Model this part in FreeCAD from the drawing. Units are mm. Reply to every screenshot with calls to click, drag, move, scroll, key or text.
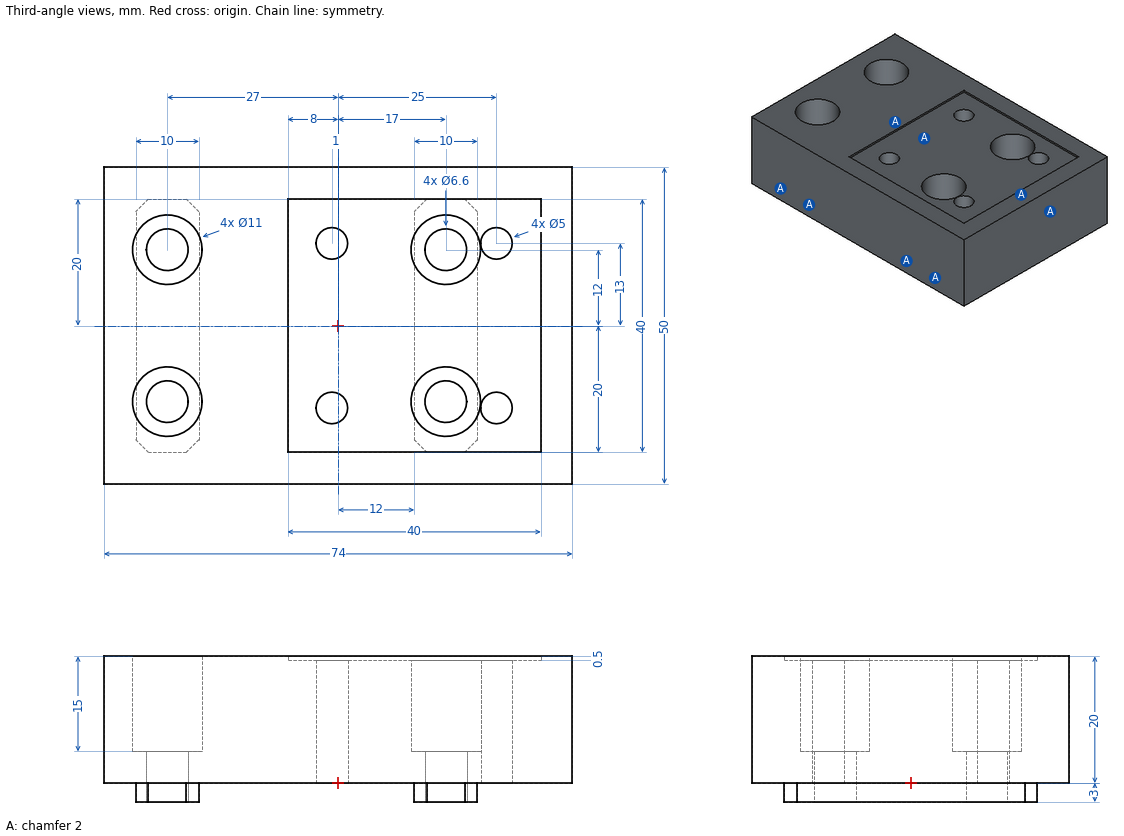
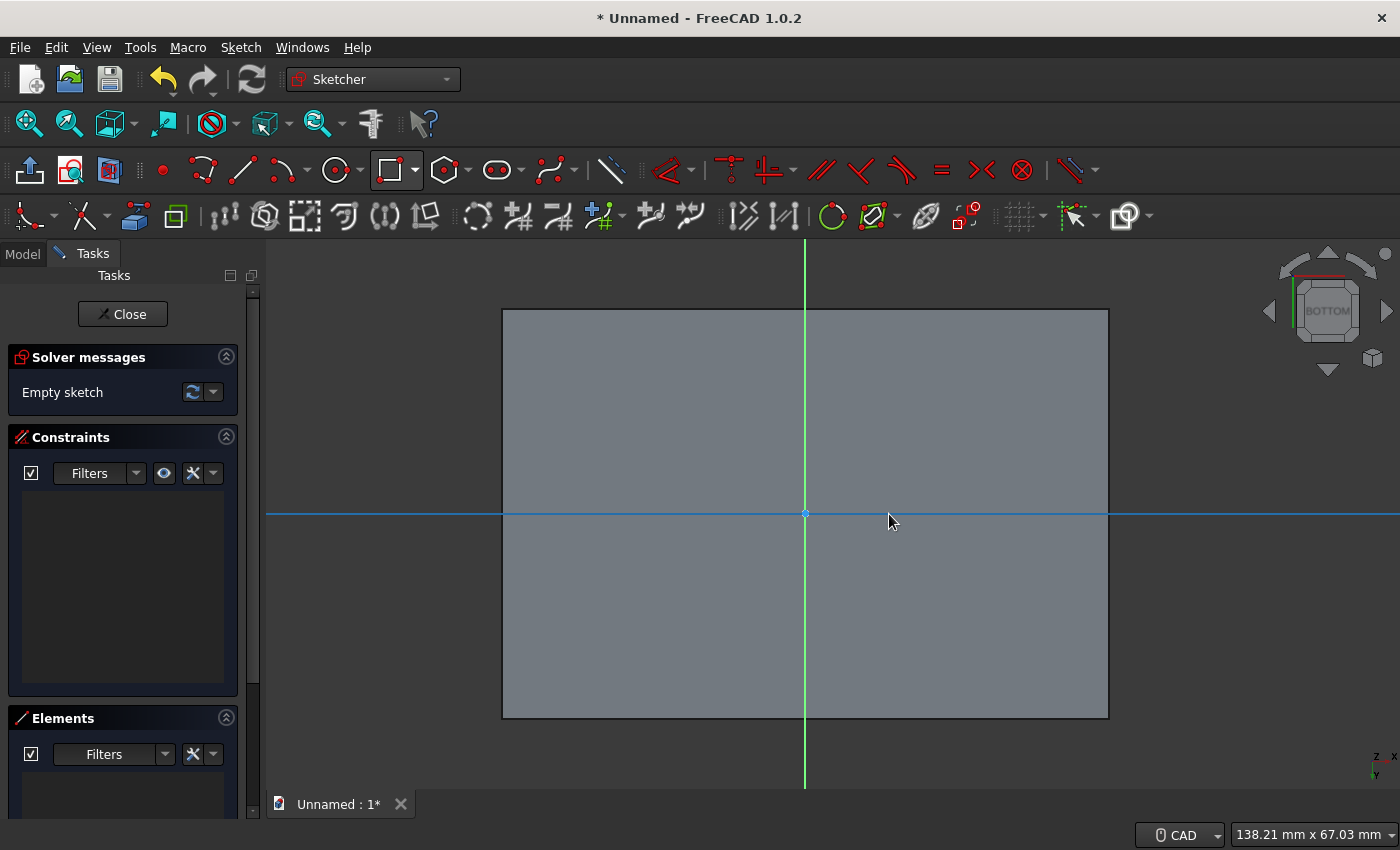
click(390, 170)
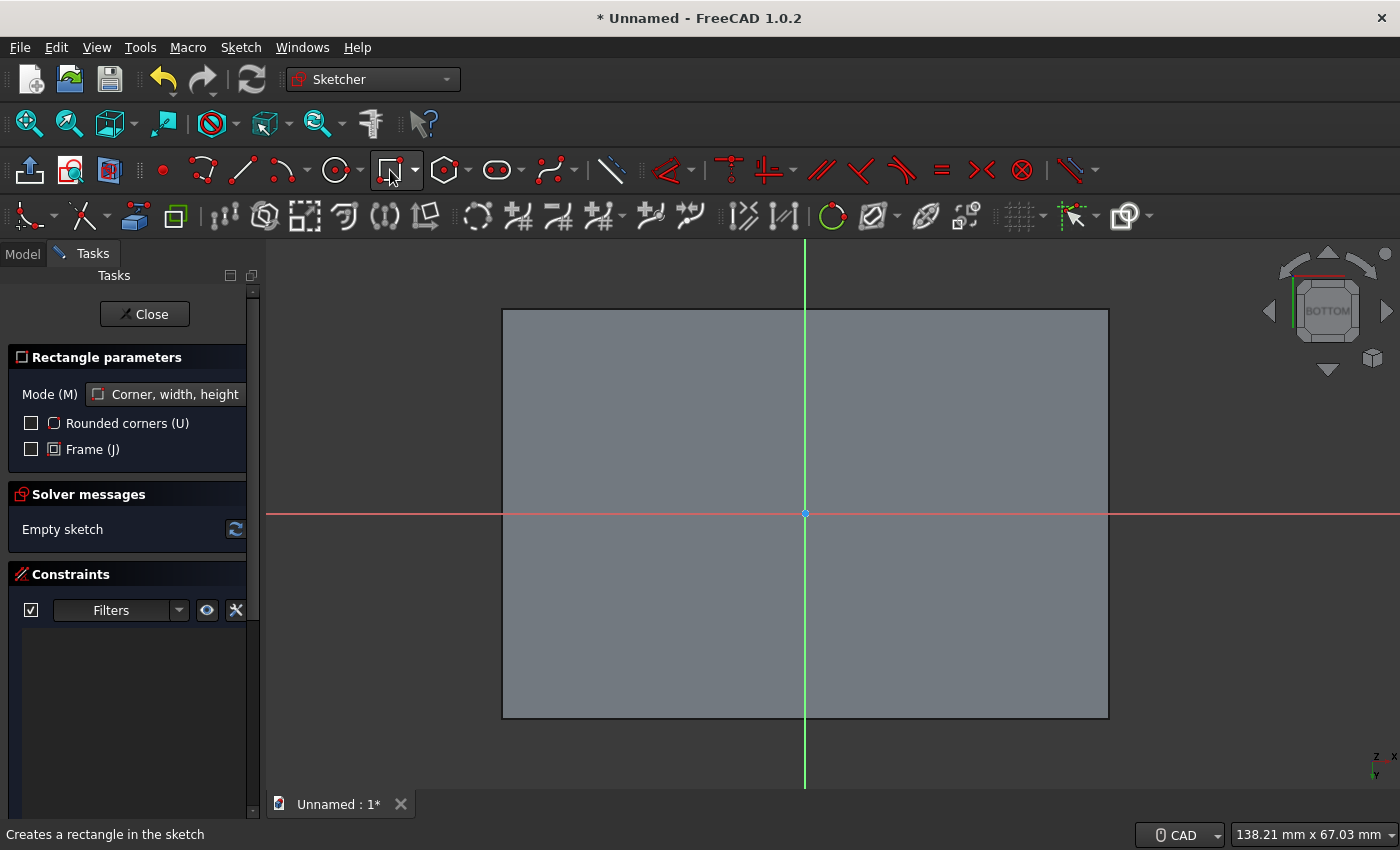
click(904, 350)
move(986, 678)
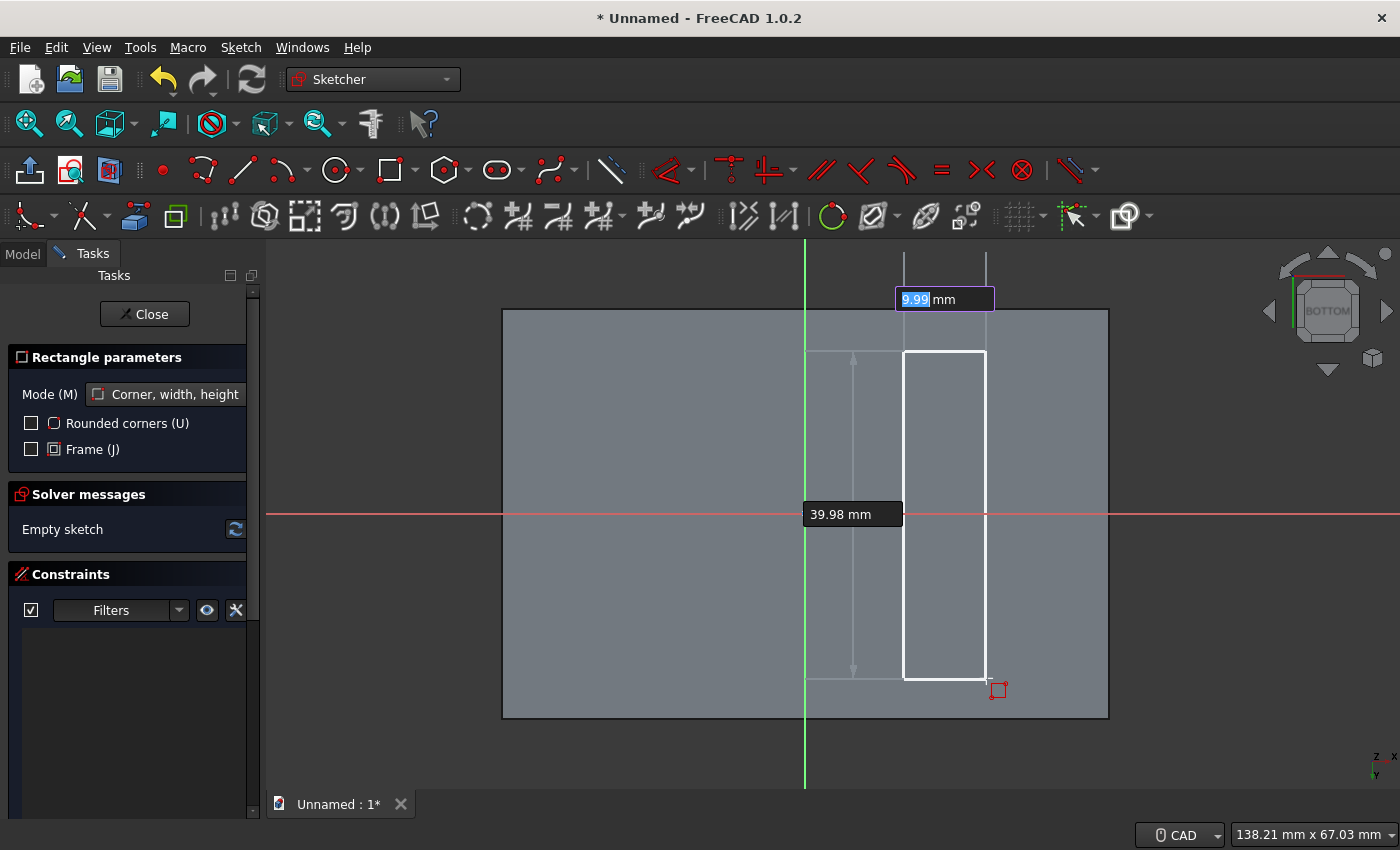
text(10)
key(Tab)
text(40)
key(Return)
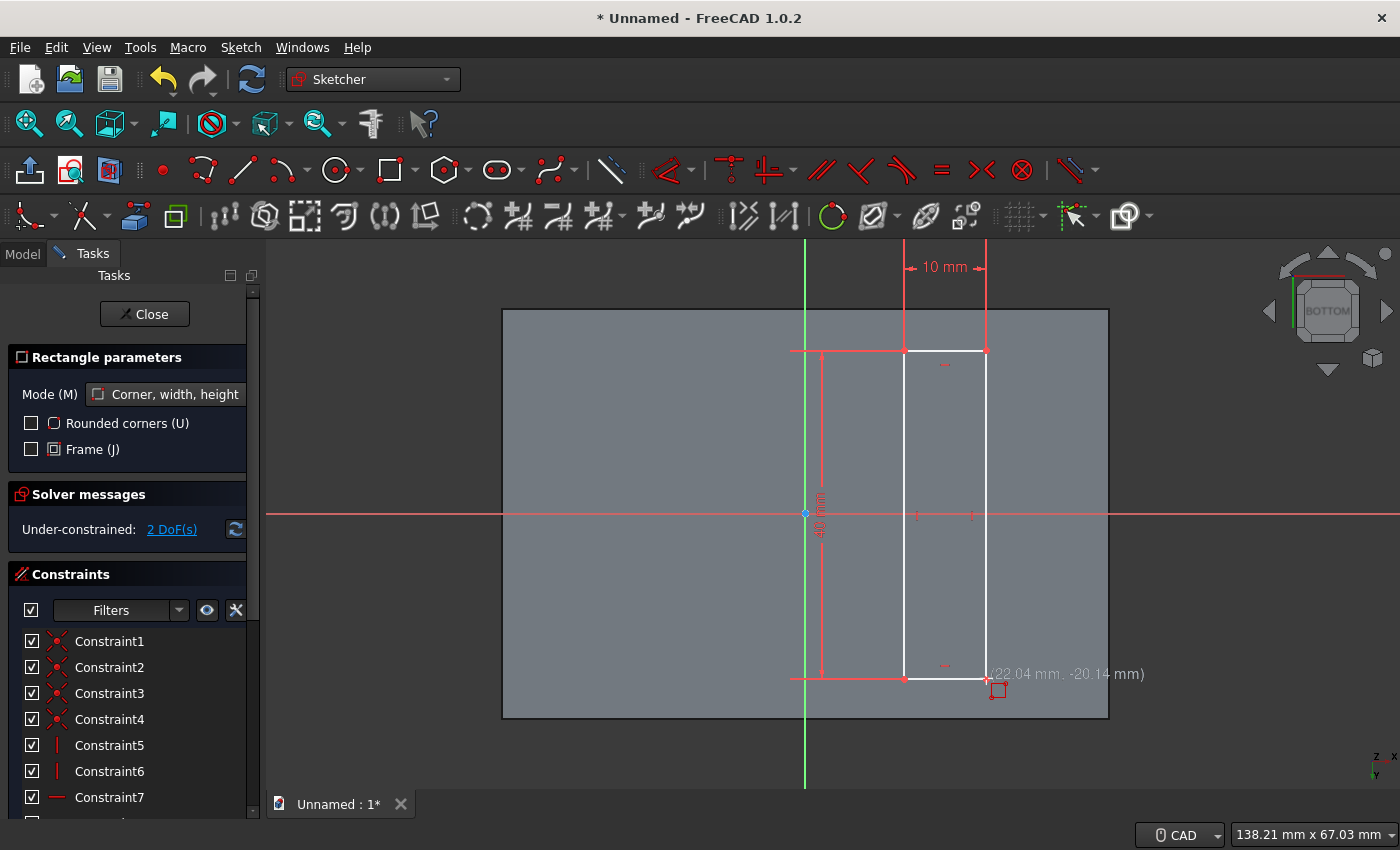
click(543, 350)
move(625, 678)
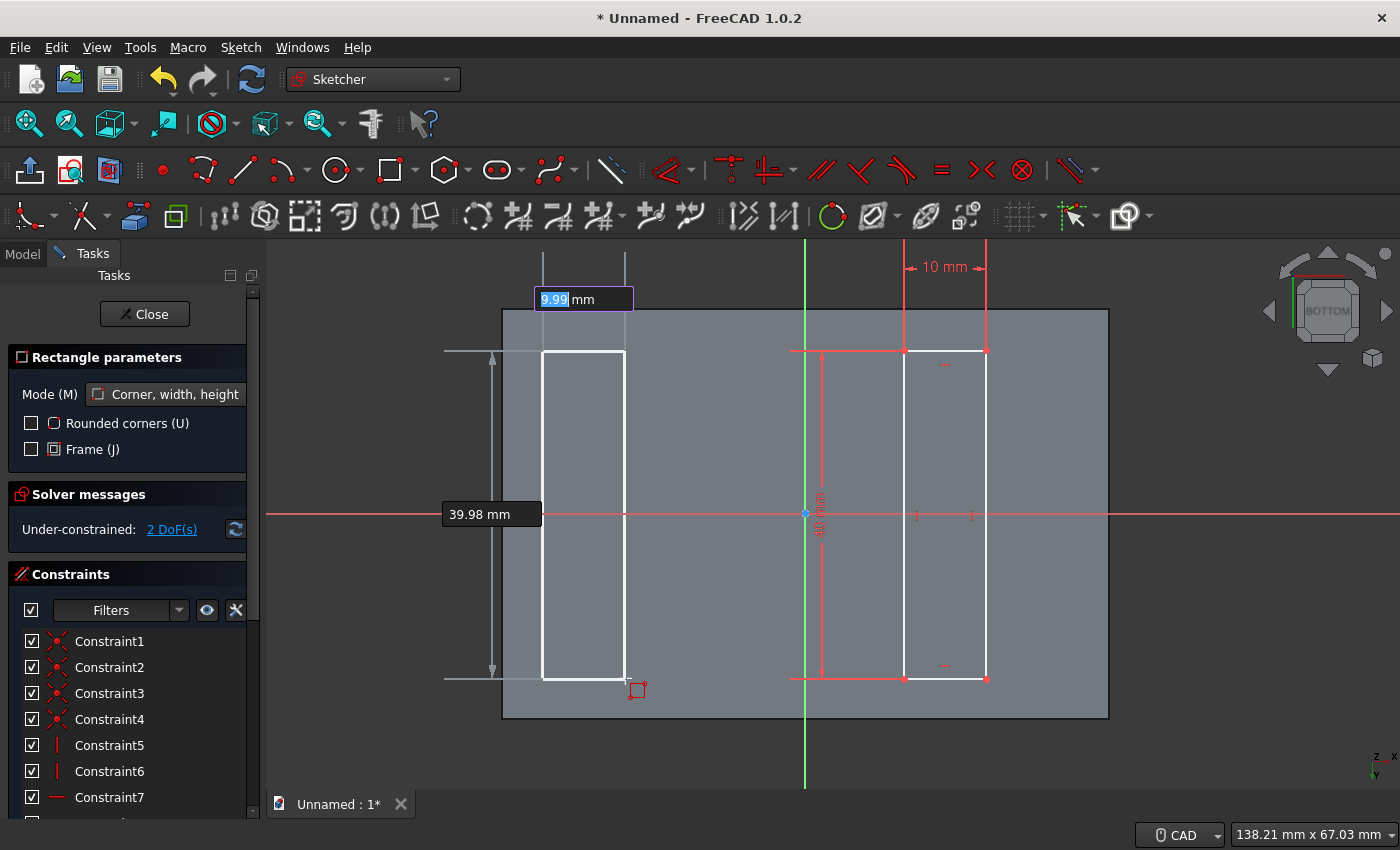
text(10)
key(Tab)
text(40)
key(Return)
key(Escape)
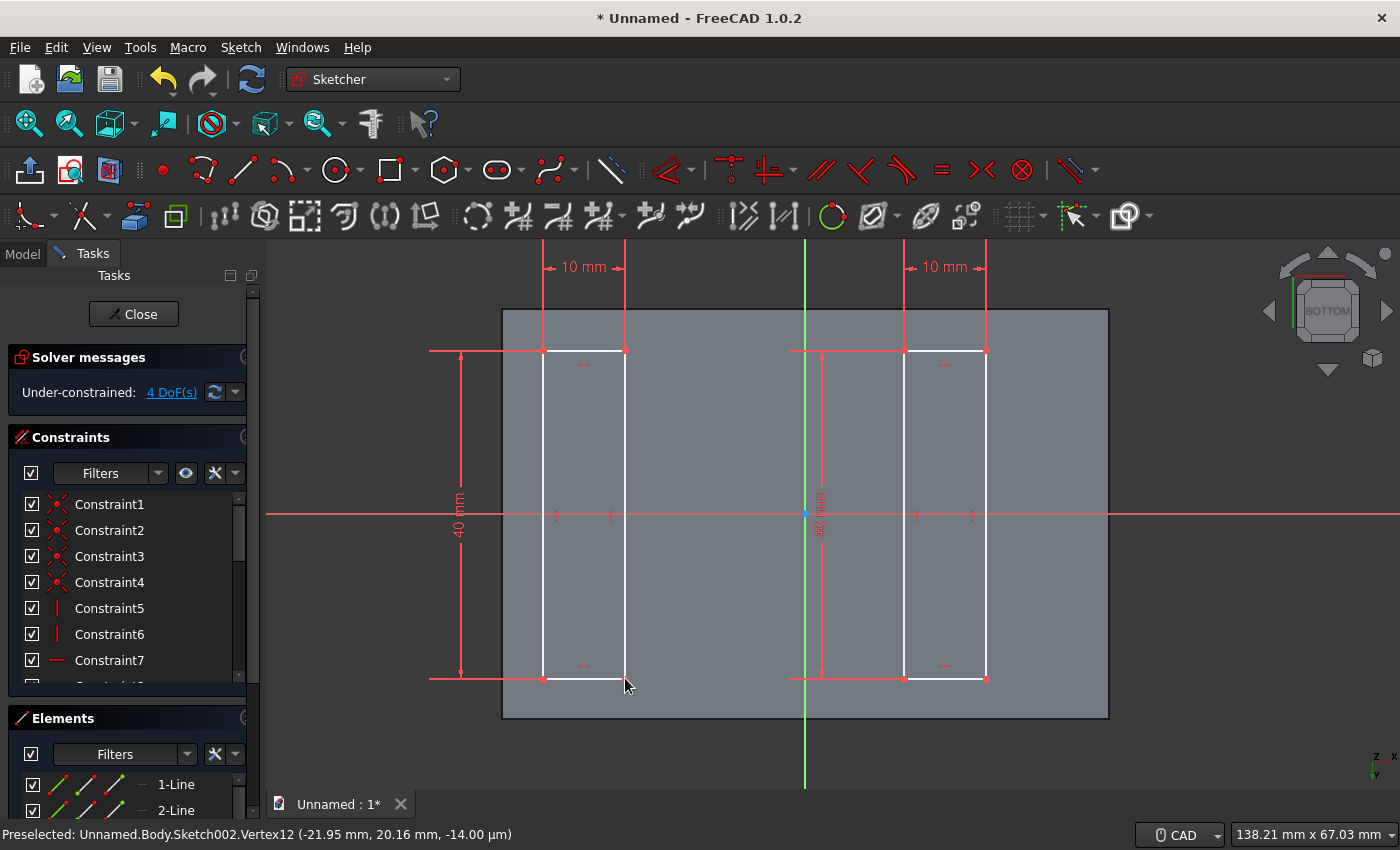
click(986, 679)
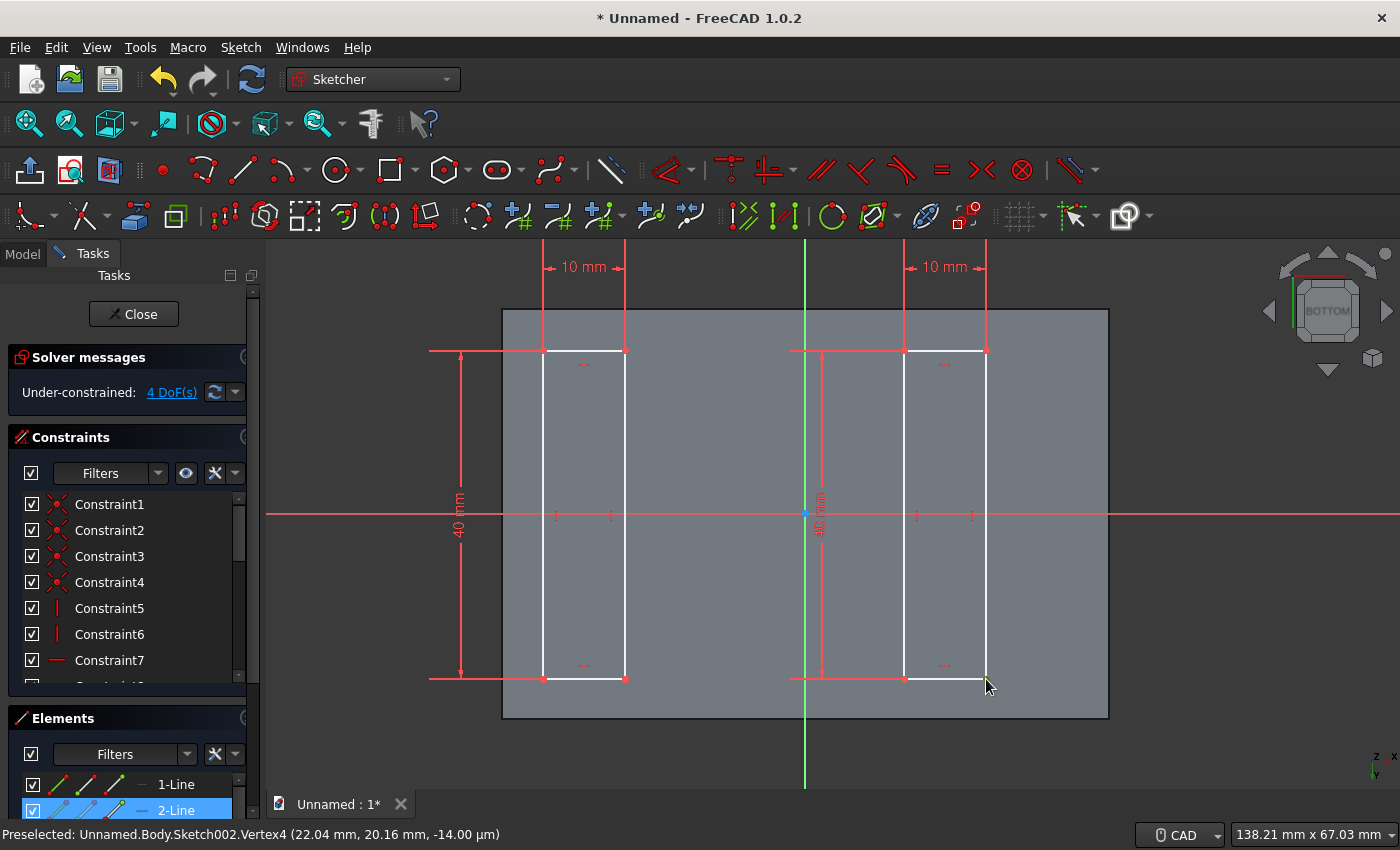
click(625, 679)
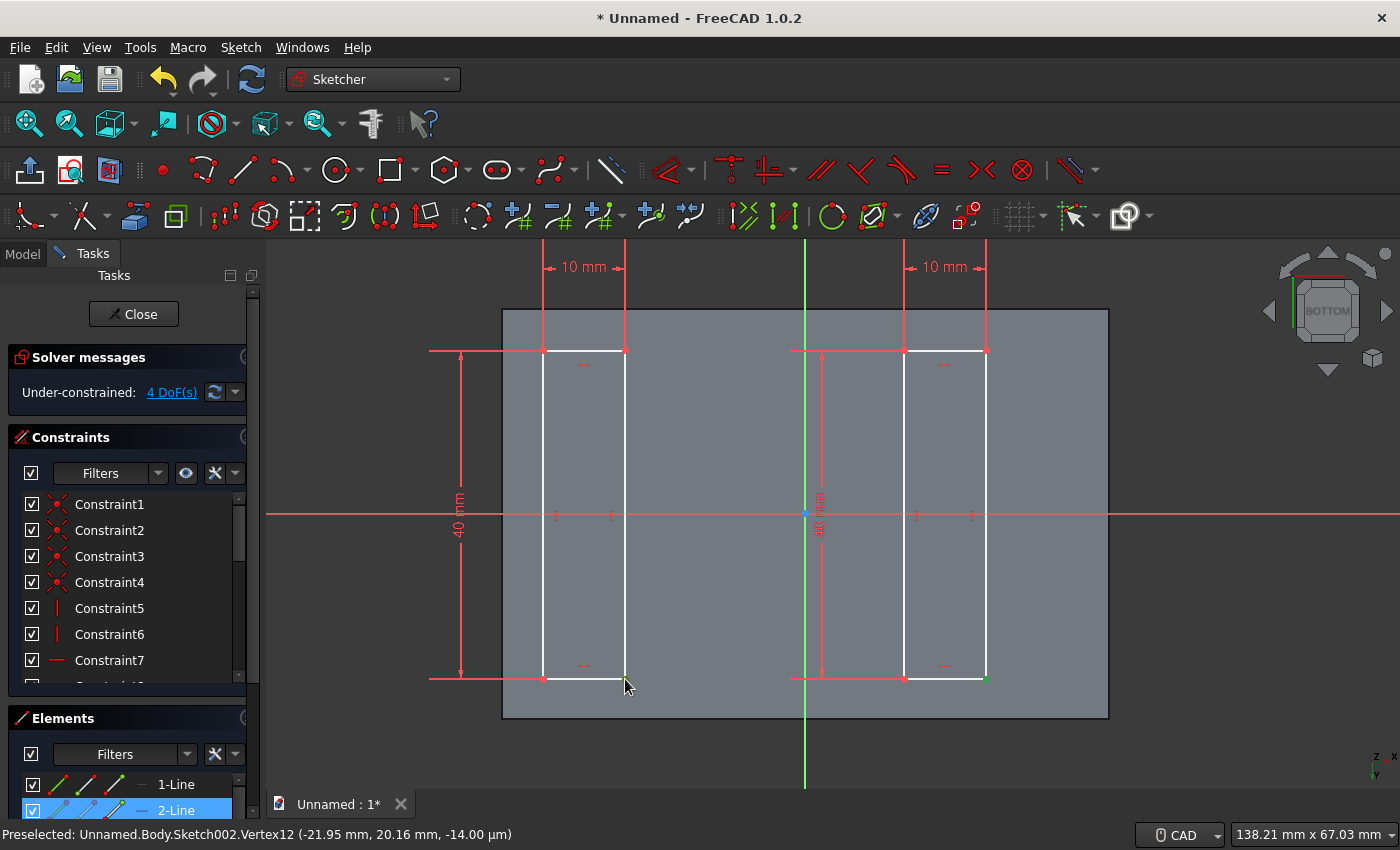
click(805, 726)